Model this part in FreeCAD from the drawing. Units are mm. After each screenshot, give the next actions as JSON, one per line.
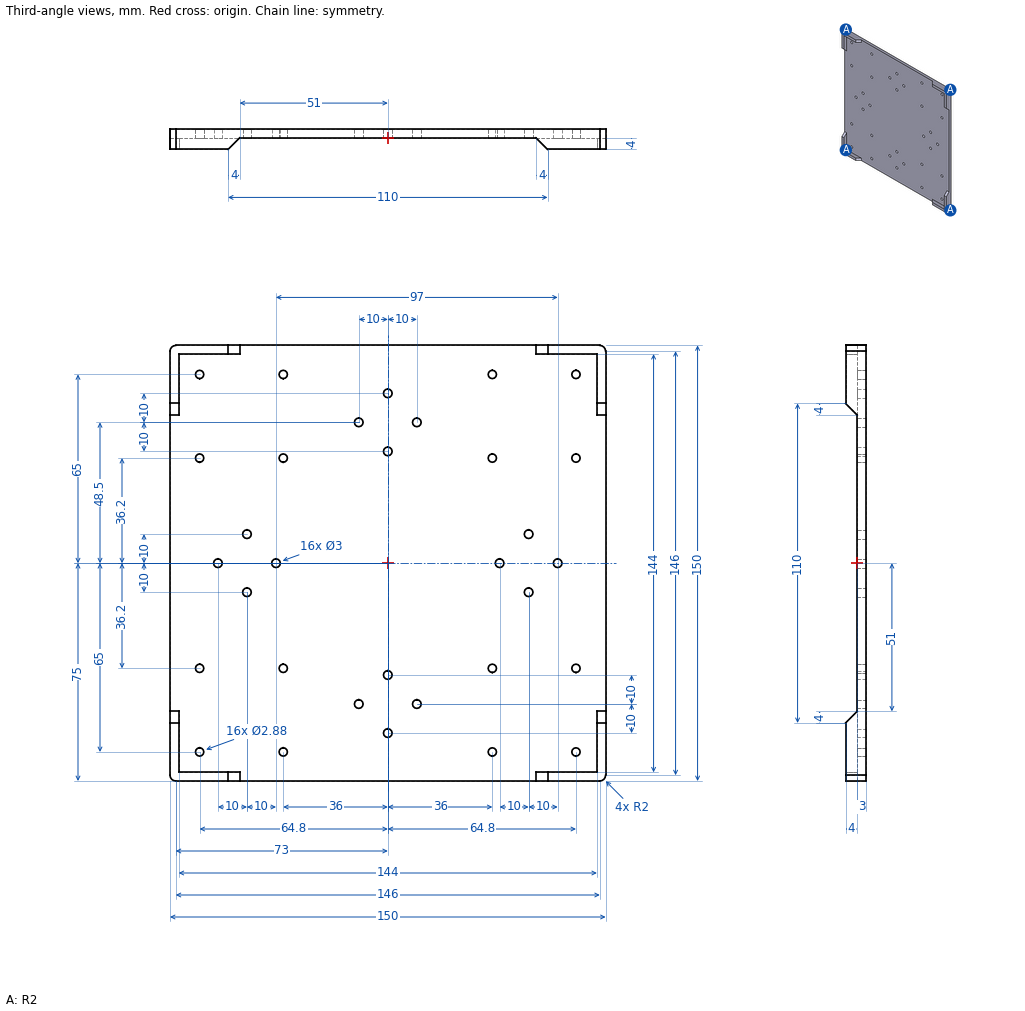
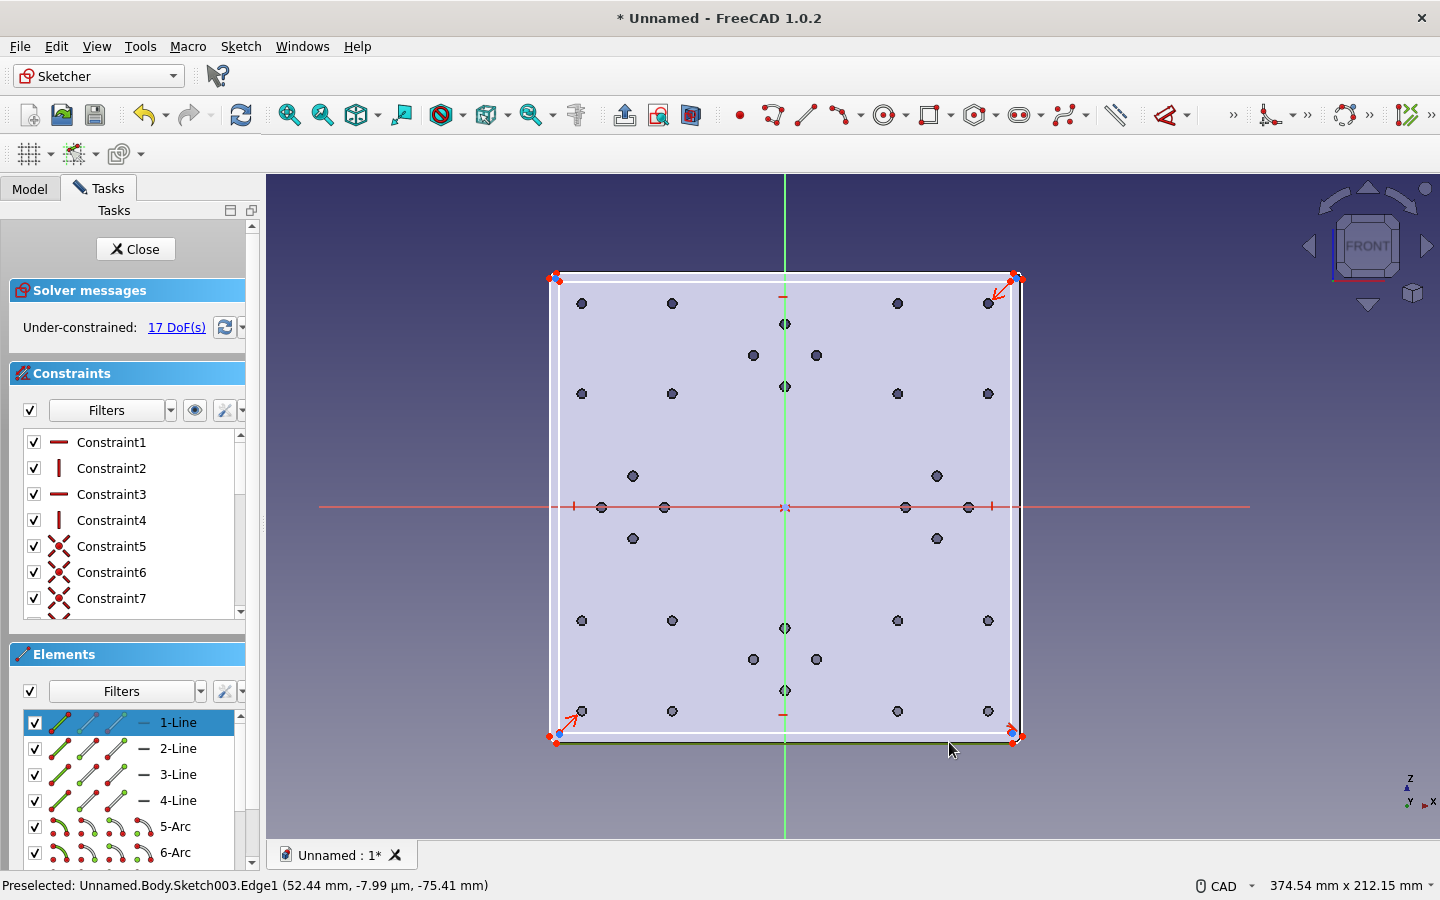
{"action": "scroll", "coordinate": [551, 739], "scroll_direction": "up", "scroll_amount": 8}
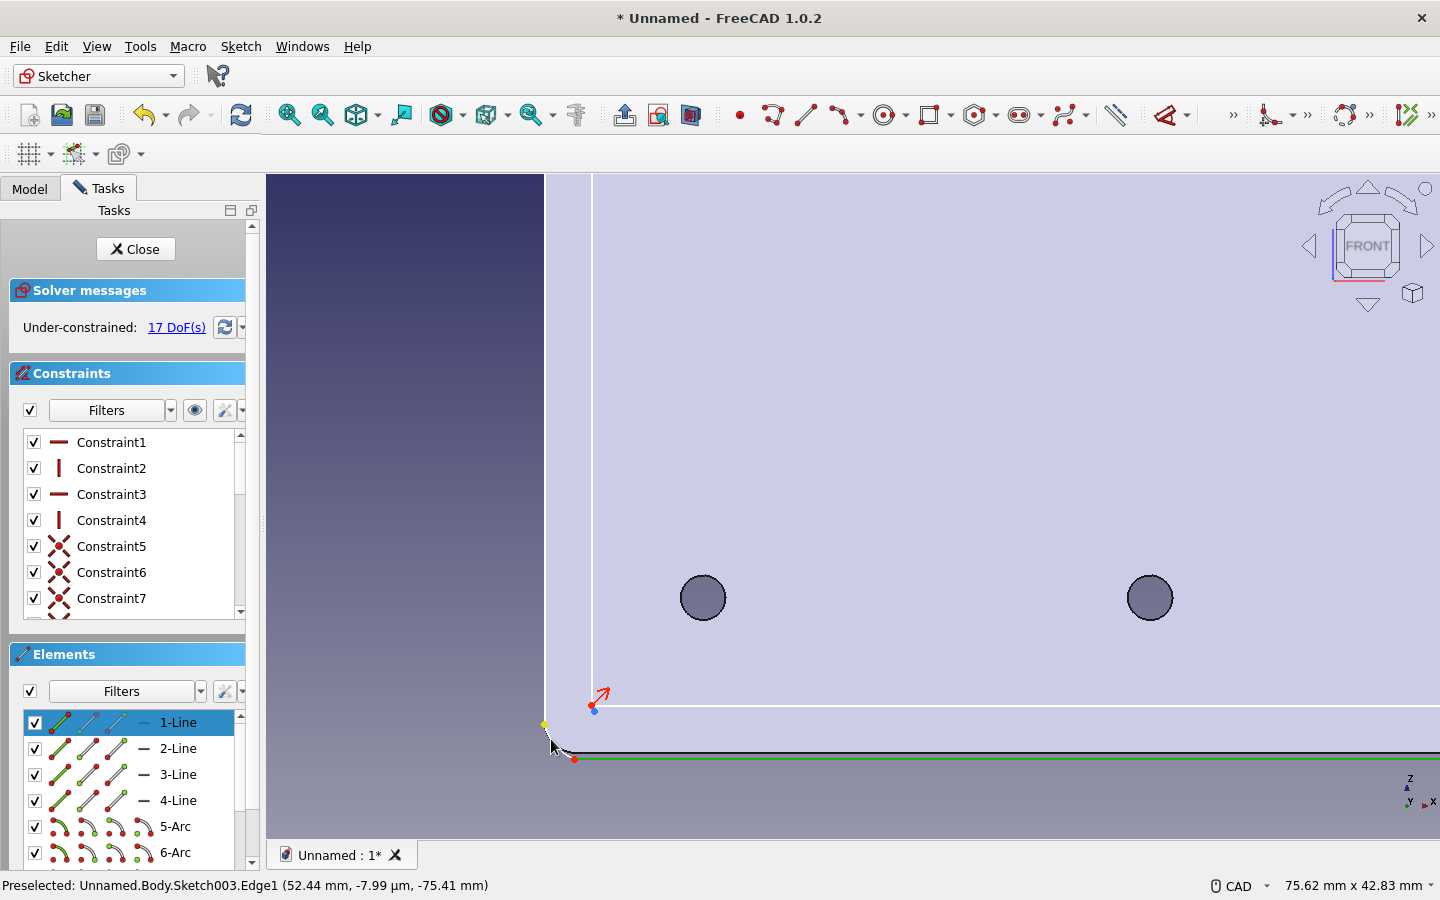
{"action": "left_click", "coordinate": [550, 738]}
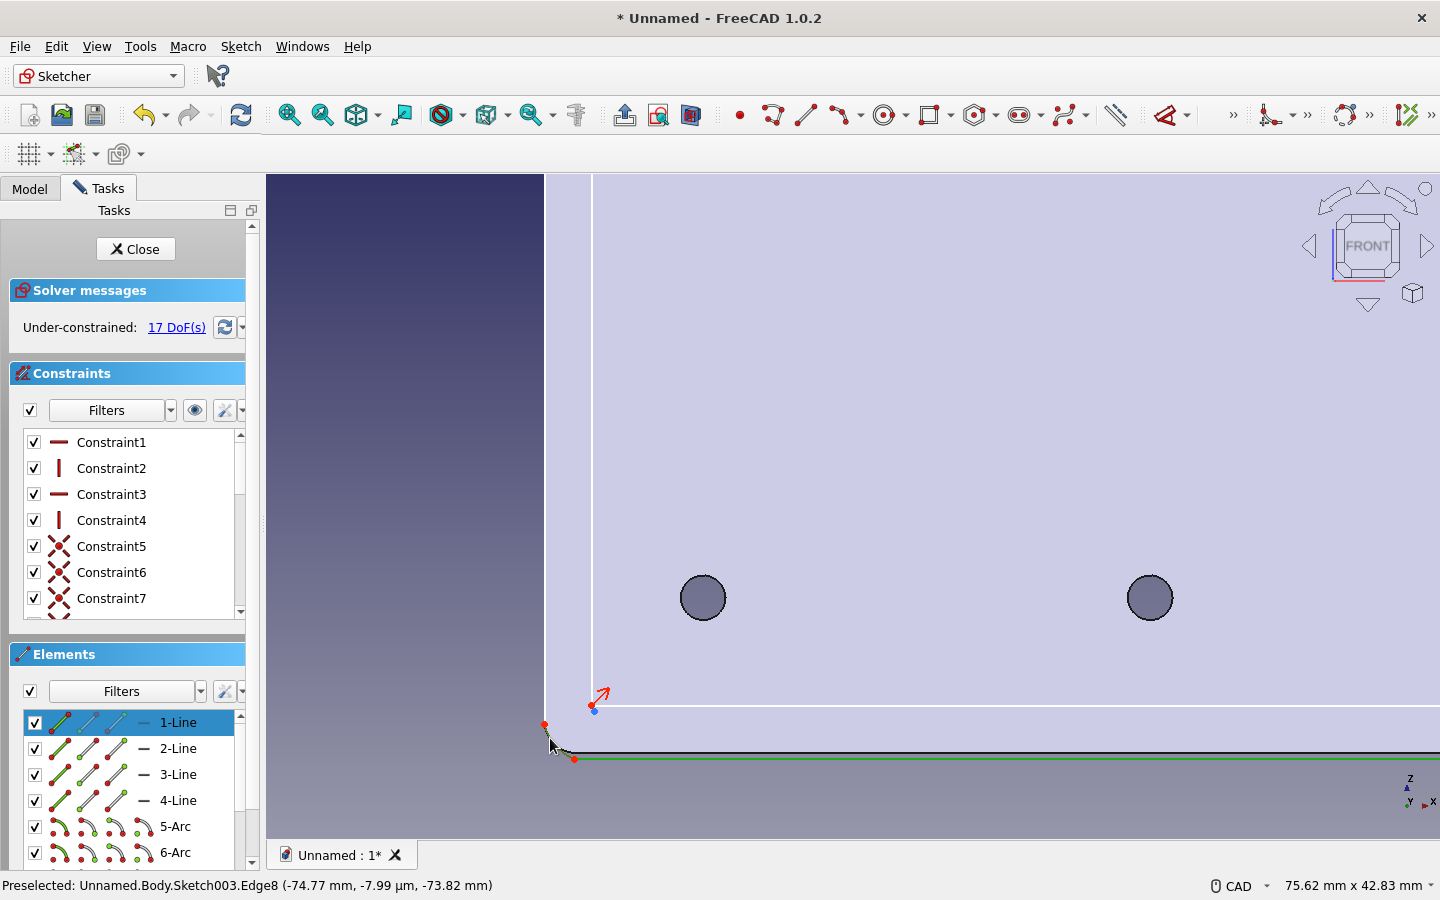
{"action": "key", "text": "t"}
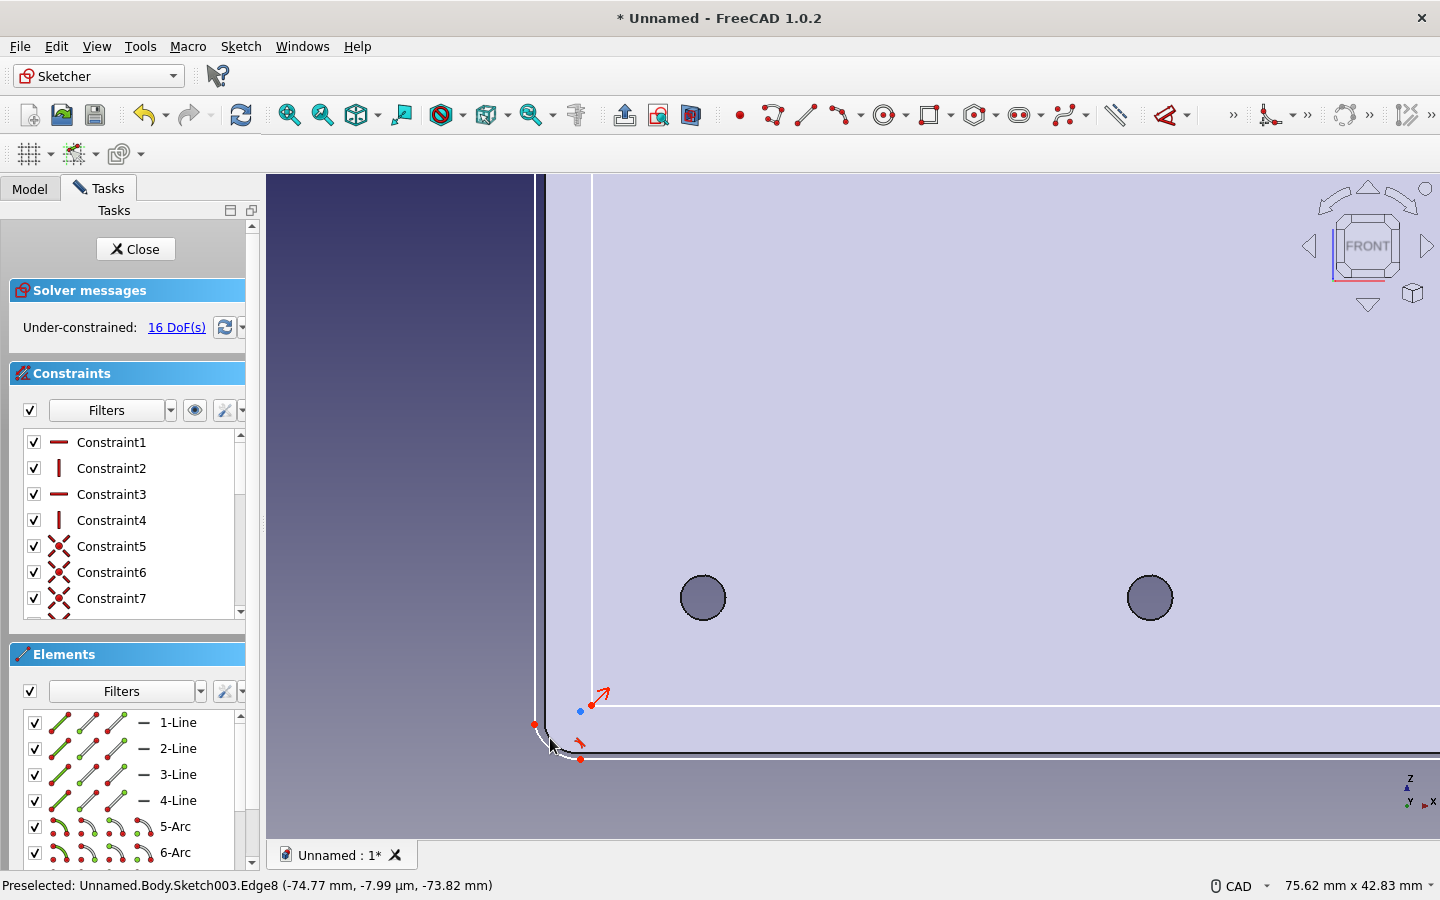
{"action": "scroll", "coordinate": [551, 739], "scroll_direction": "down", "scroll_amount": 8}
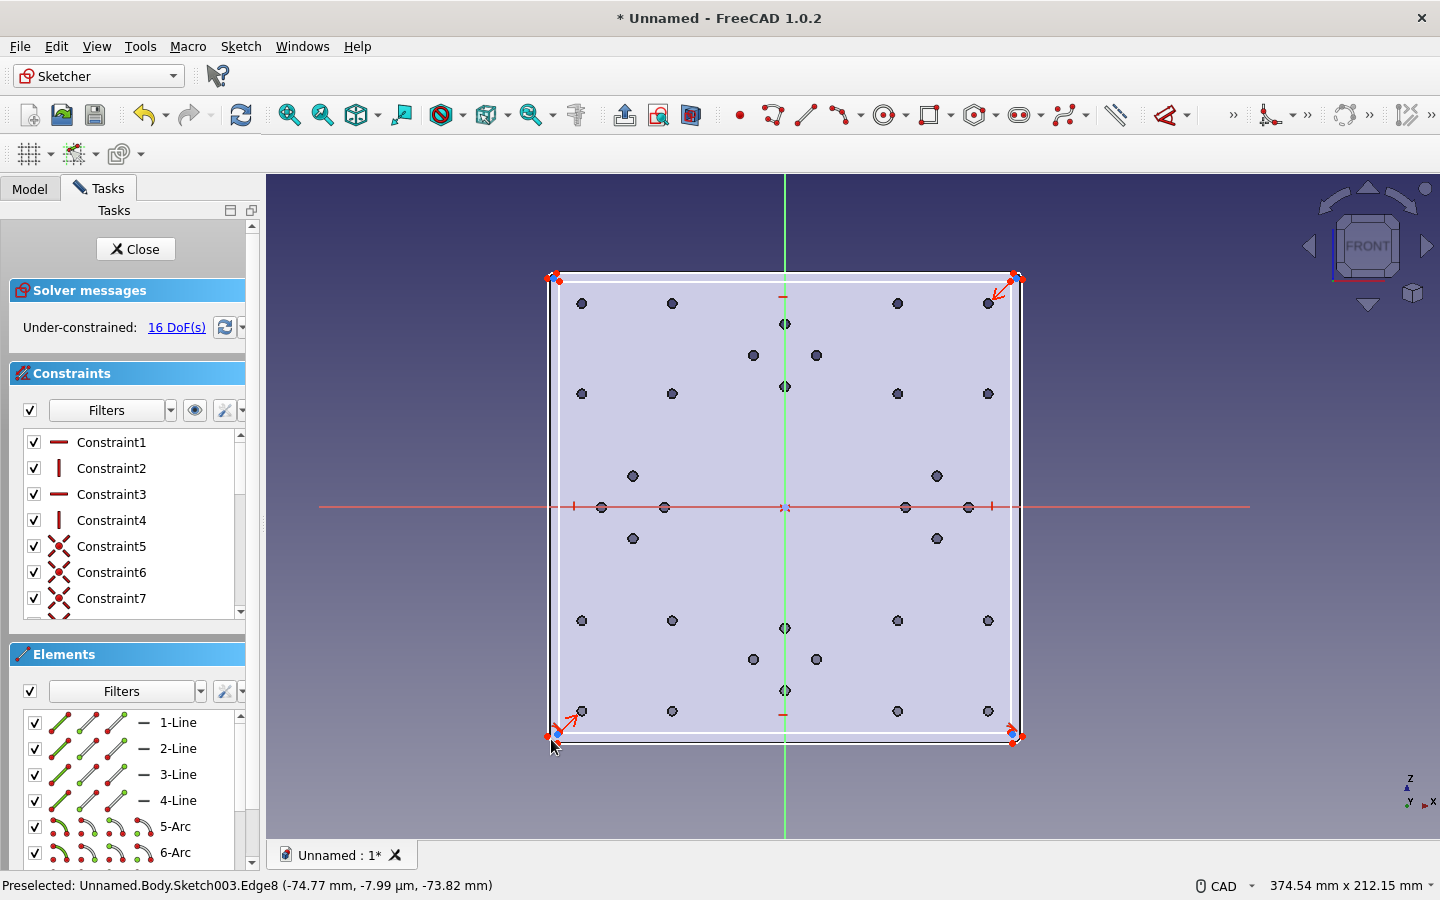
{"action": "left_click", "coordinate": [1022, 600]}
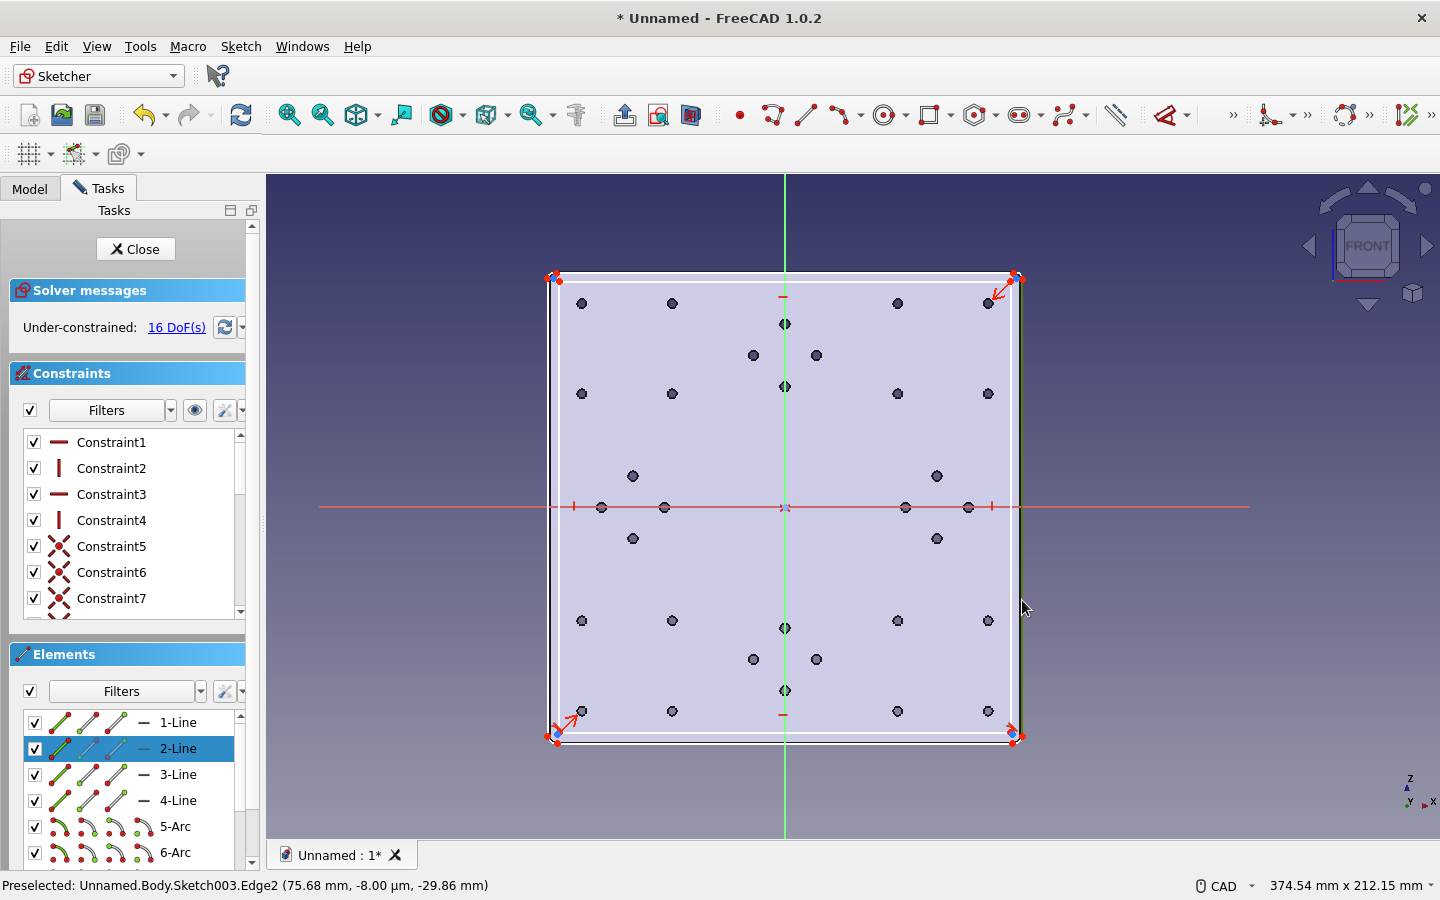
{"action": "scroll", "coordinate": [1019, 742], "scroll_direction": "up", "scroll_amount": 5}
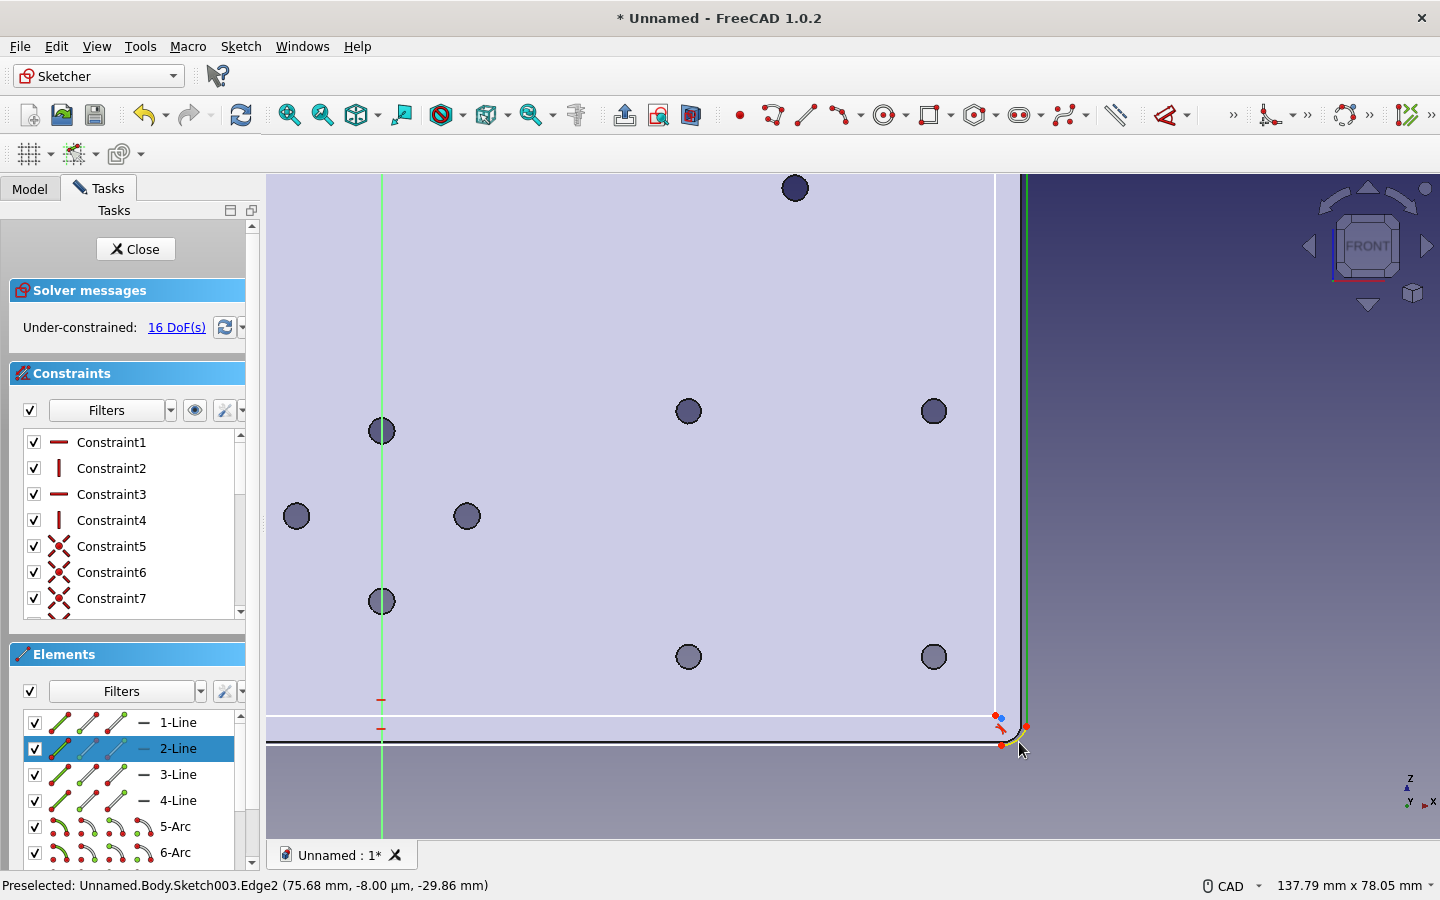
{"action": "left_click", "coordinate": [1017, 740]}